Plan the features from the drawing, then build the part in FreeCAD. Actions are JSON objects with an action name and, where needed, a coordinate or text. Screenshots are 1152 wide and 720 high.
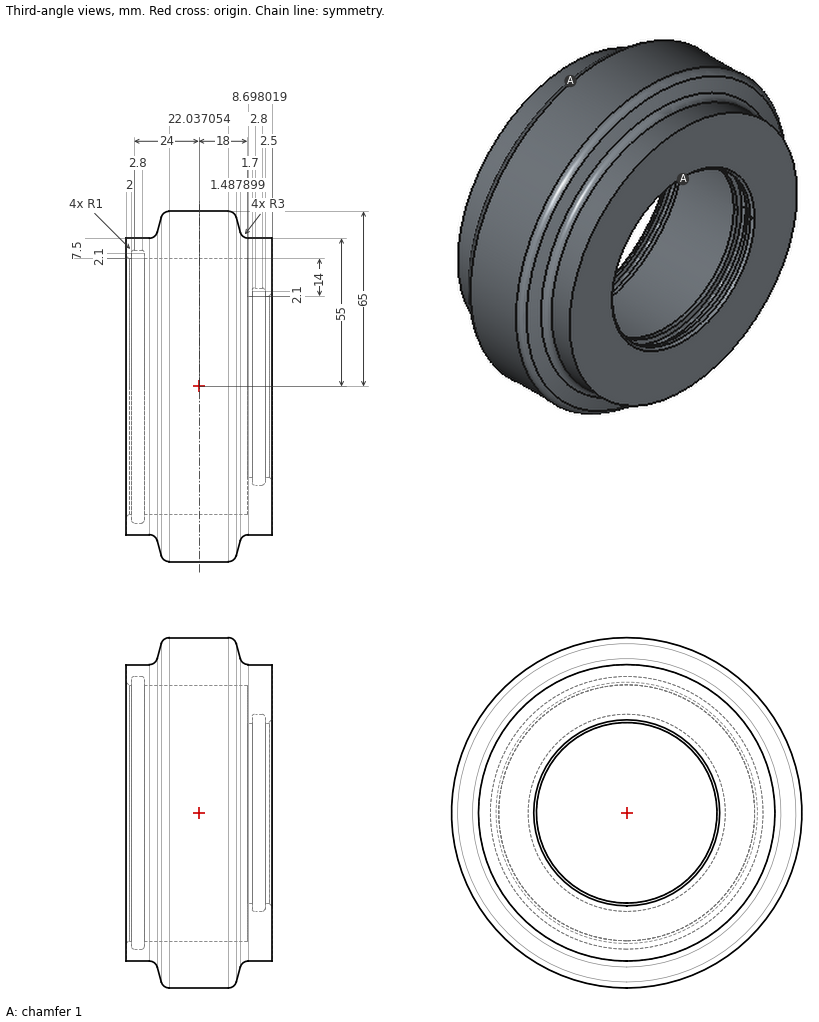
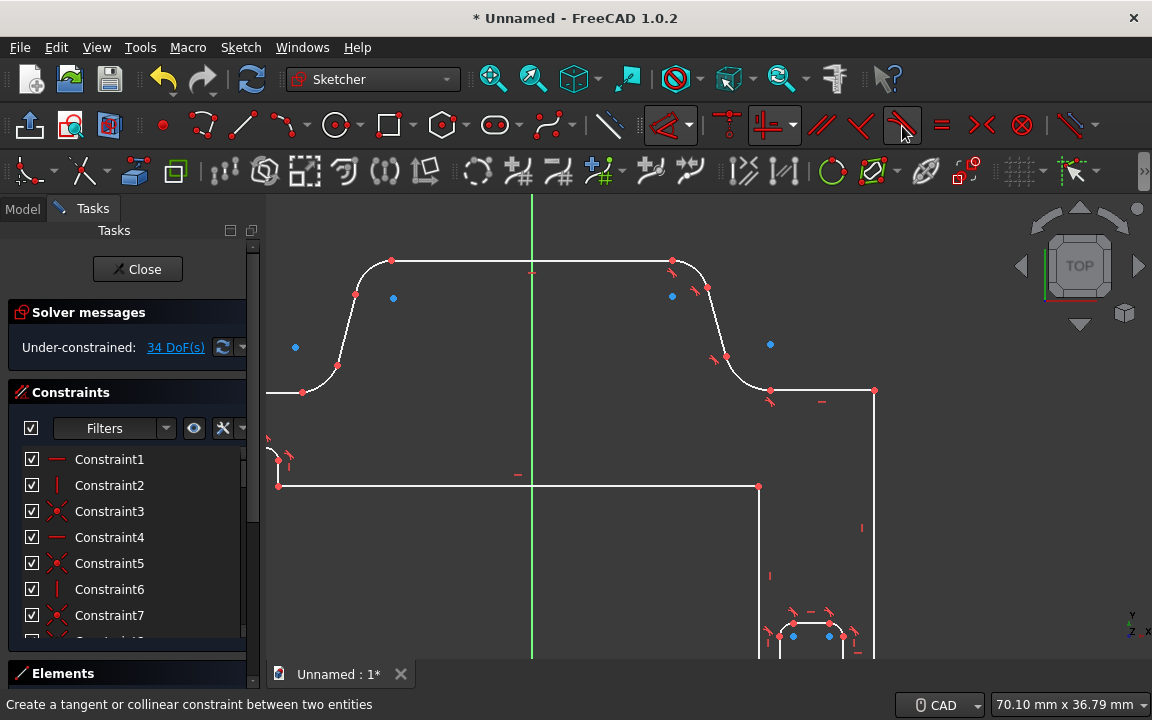
{"action": "left_click", "coordinate": [588, 261]}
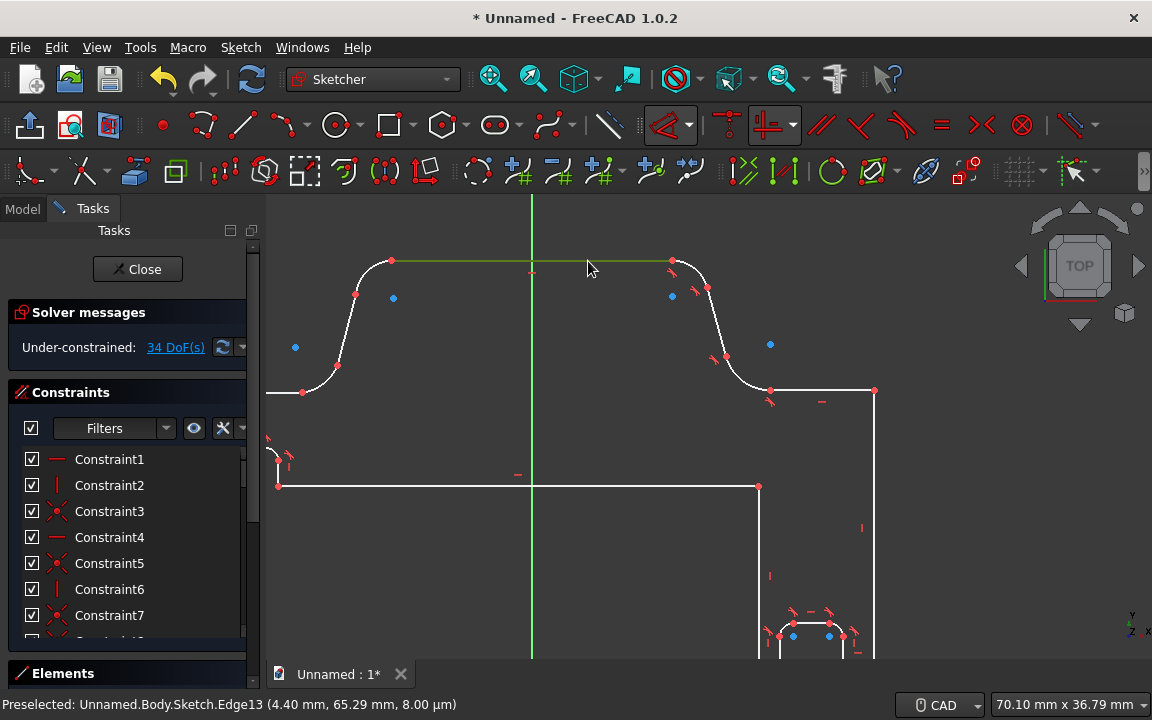
{"action": "left_click", "coordinate": [376, 265]}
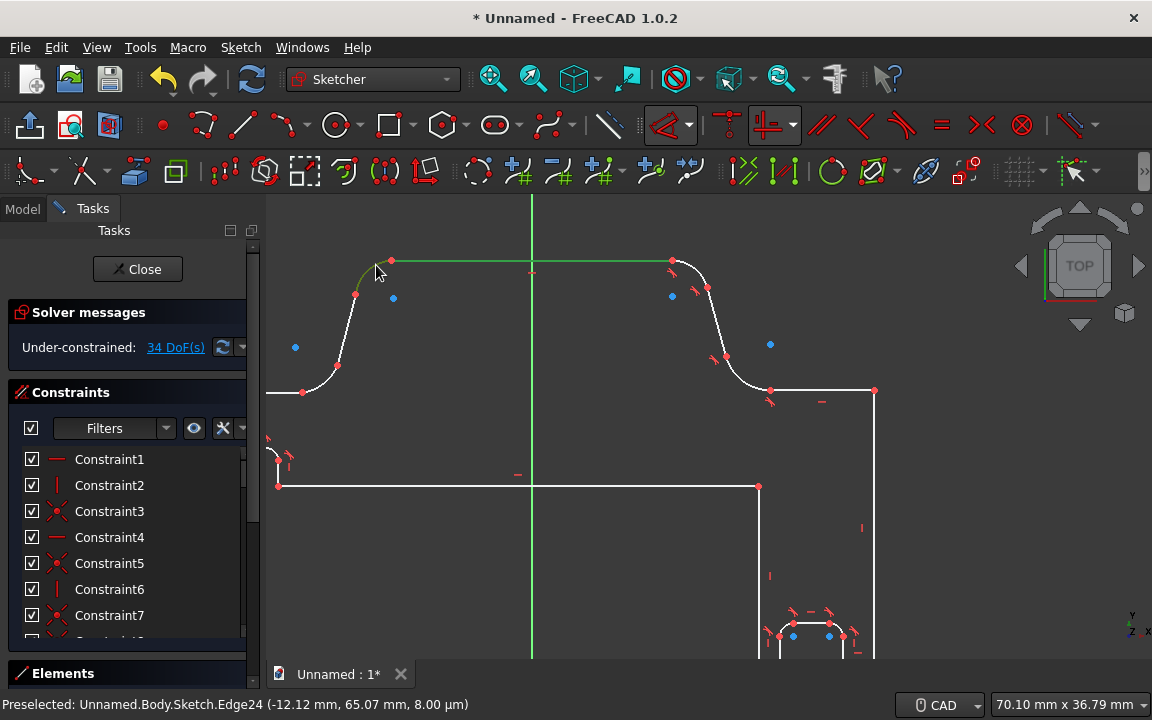
{"action": "key", "text": "t"}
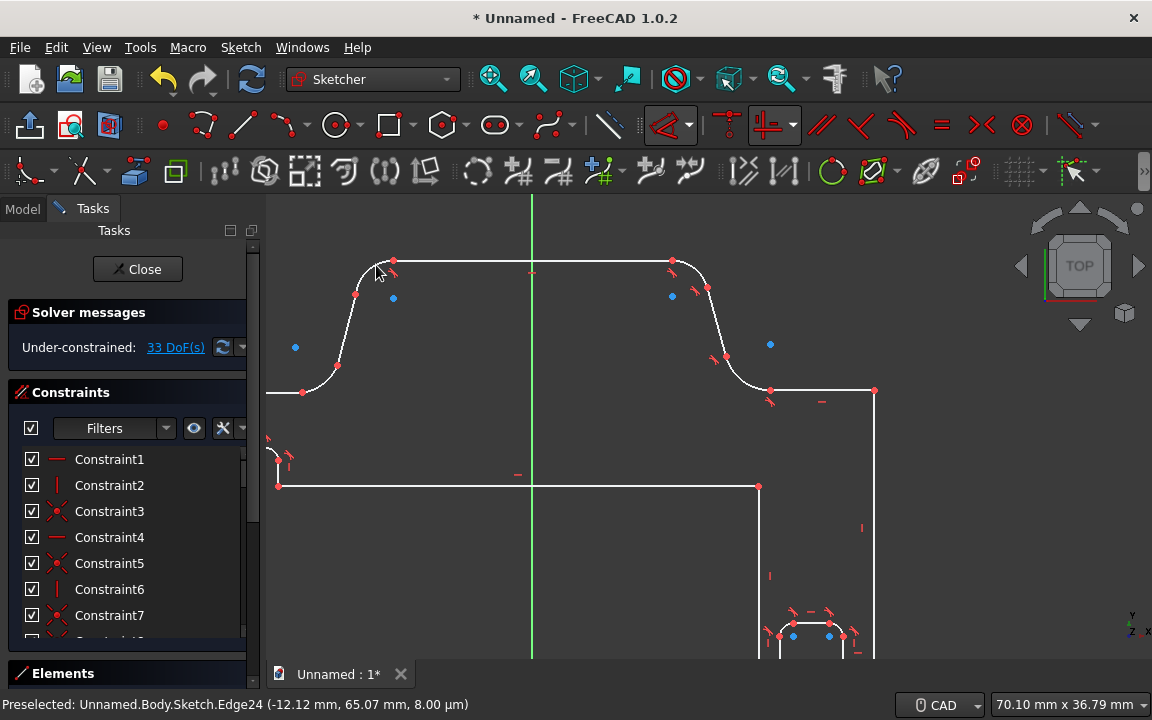
{"action": "left_click", "coordinate": [350, 316]}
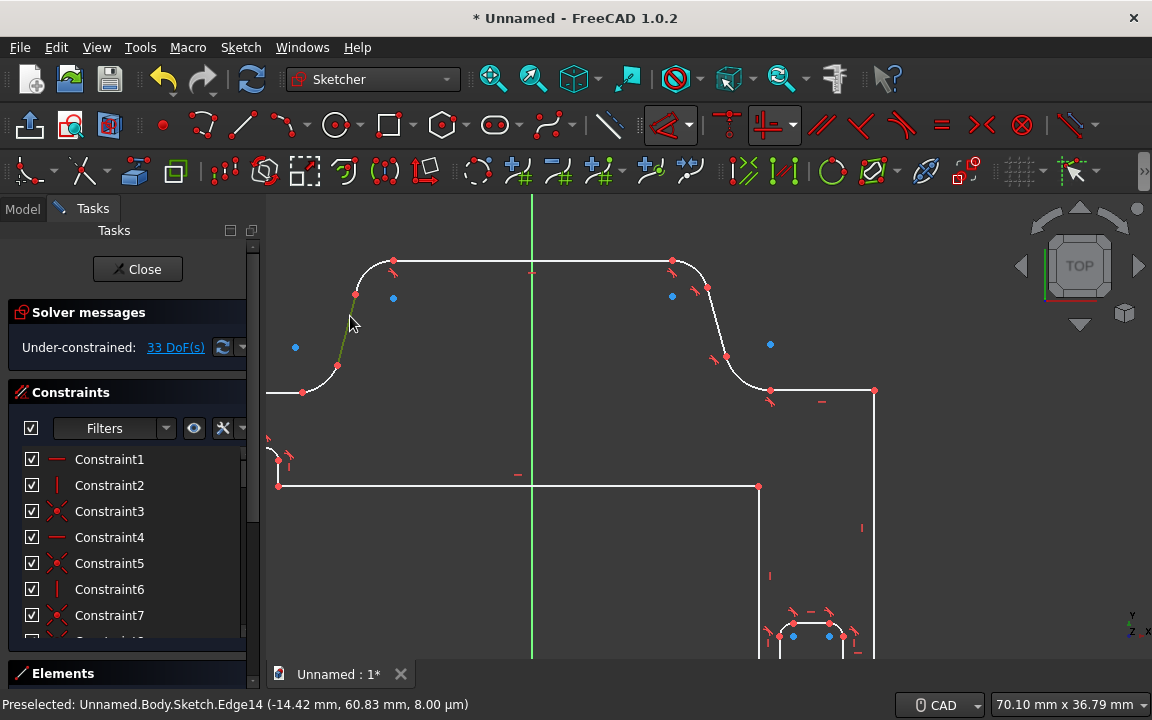
{"action": "left_click", "coordinate": [377, 264]}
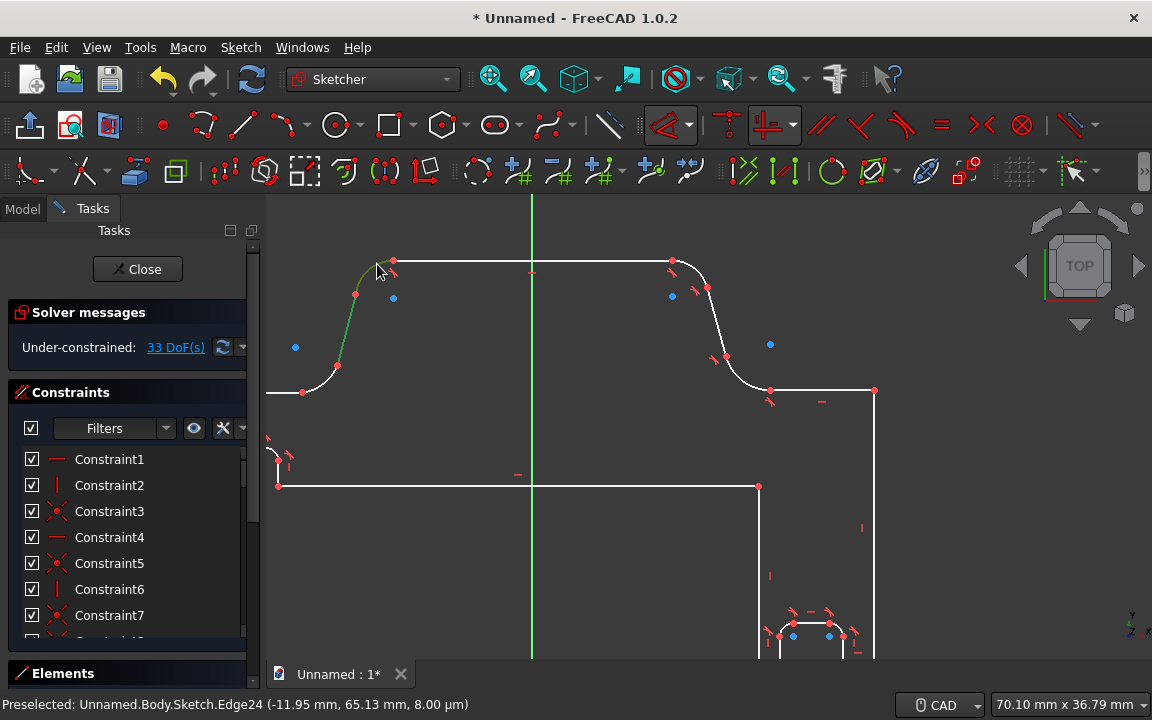
{"action": "key", "text": "t"}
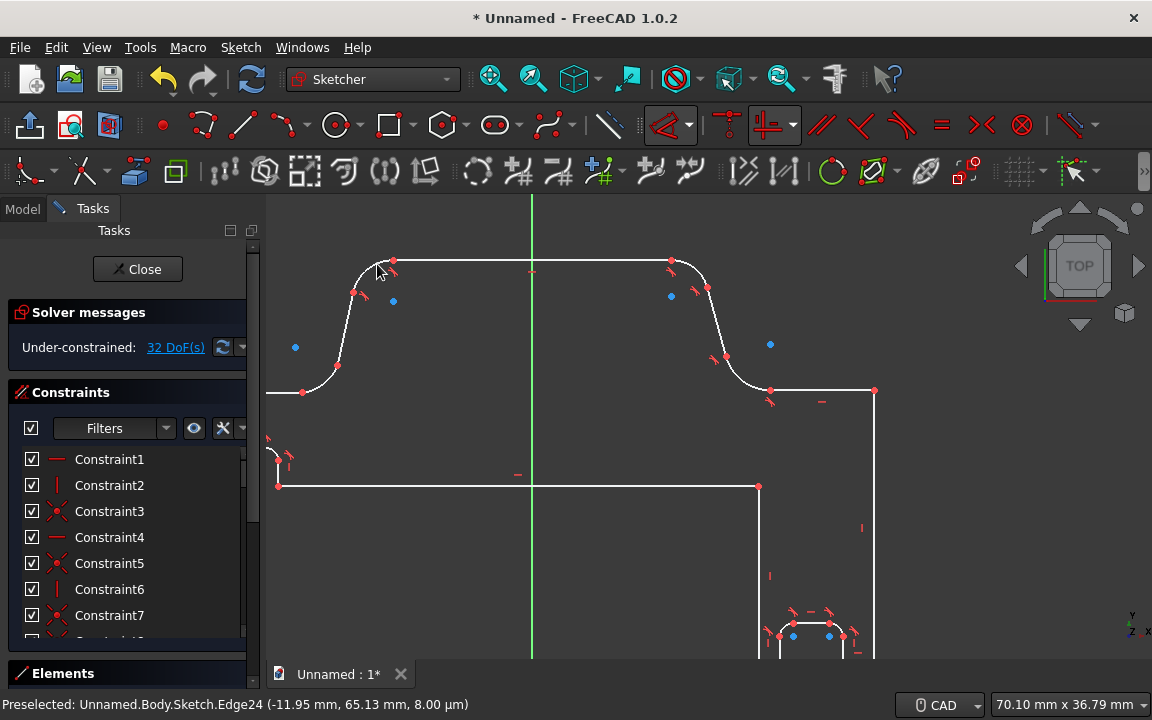
{"action": "left_click", "coordinate": [349, 315]}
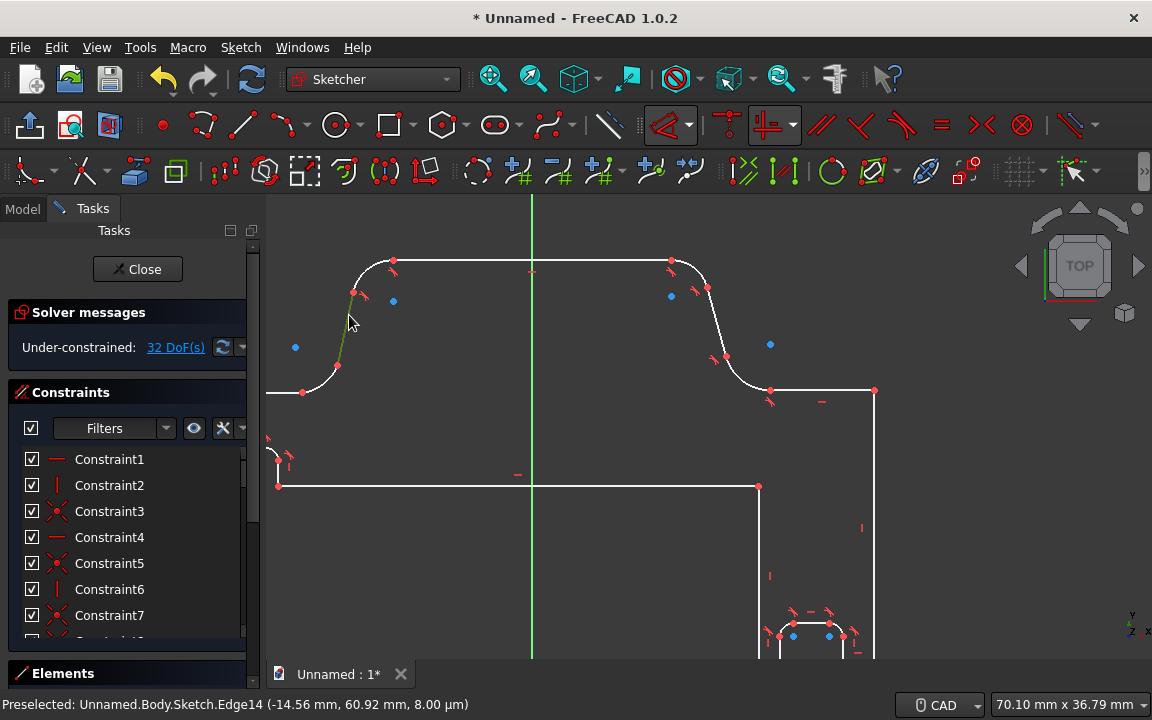
{"action": "left_click", "coordinate": [315, 389]}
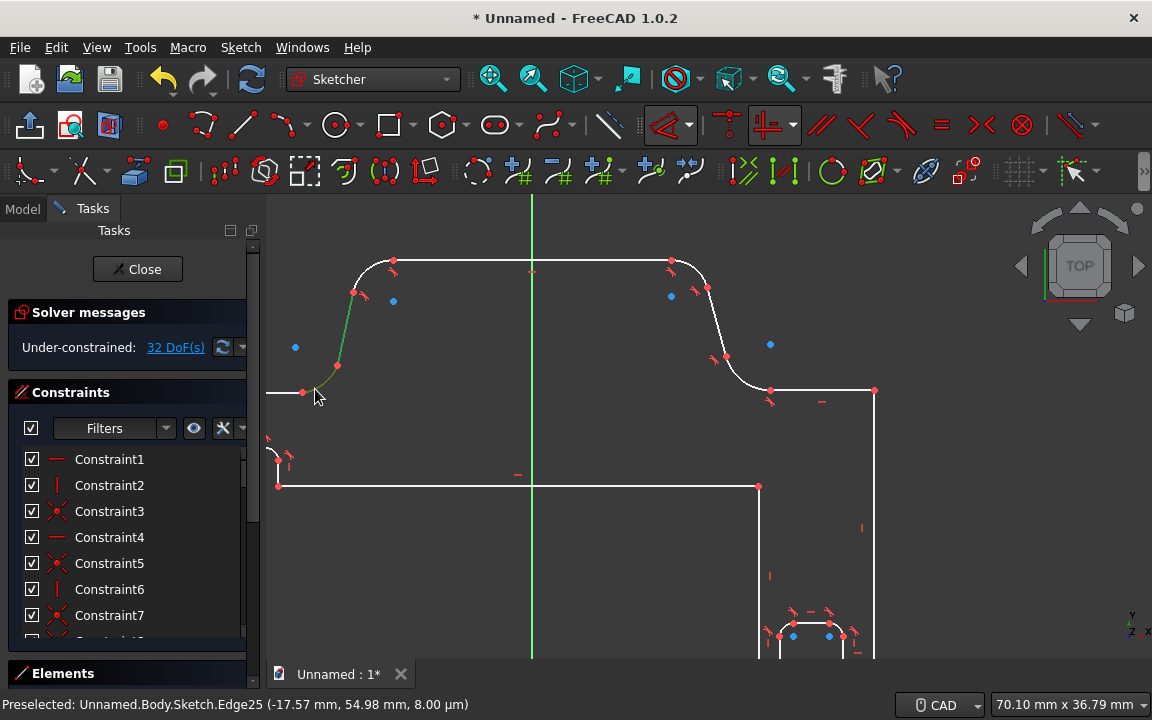
{"action": "left_click", "coordinate": [902, 126]}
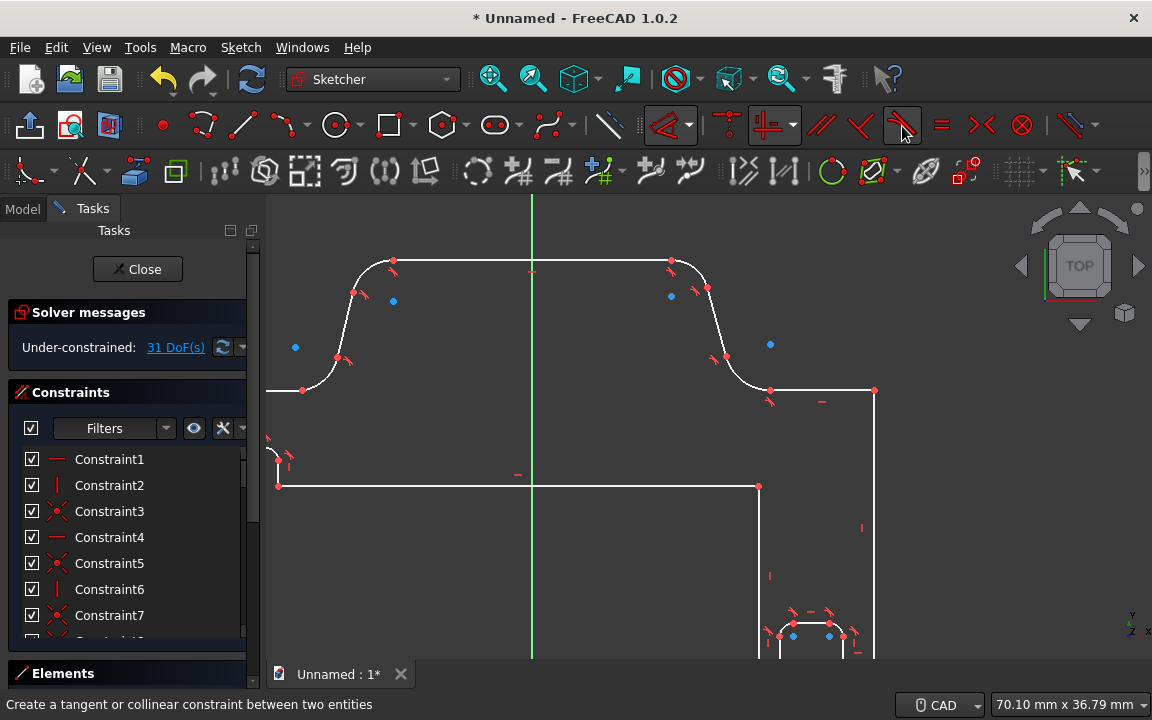
{"action": "scroll", "coordinate": [703, 282], "scroll_direction": "down", "scroll_amount": 5}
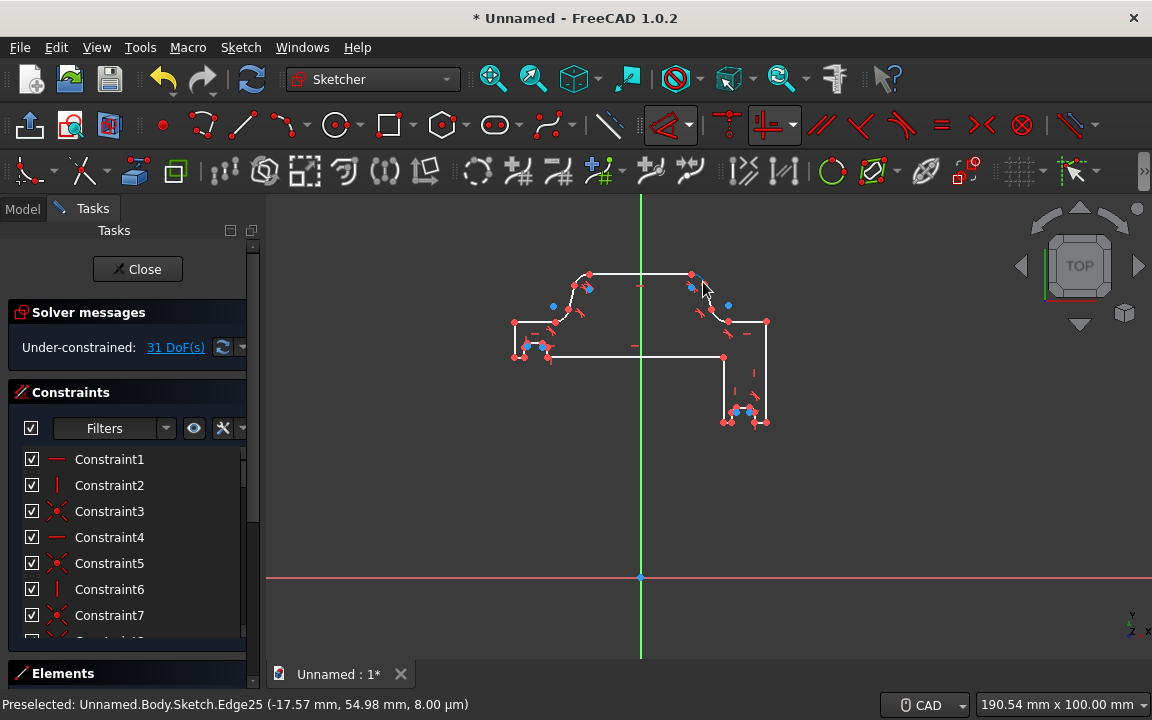
{"action": "left_click", "coordinate": [544, 322]}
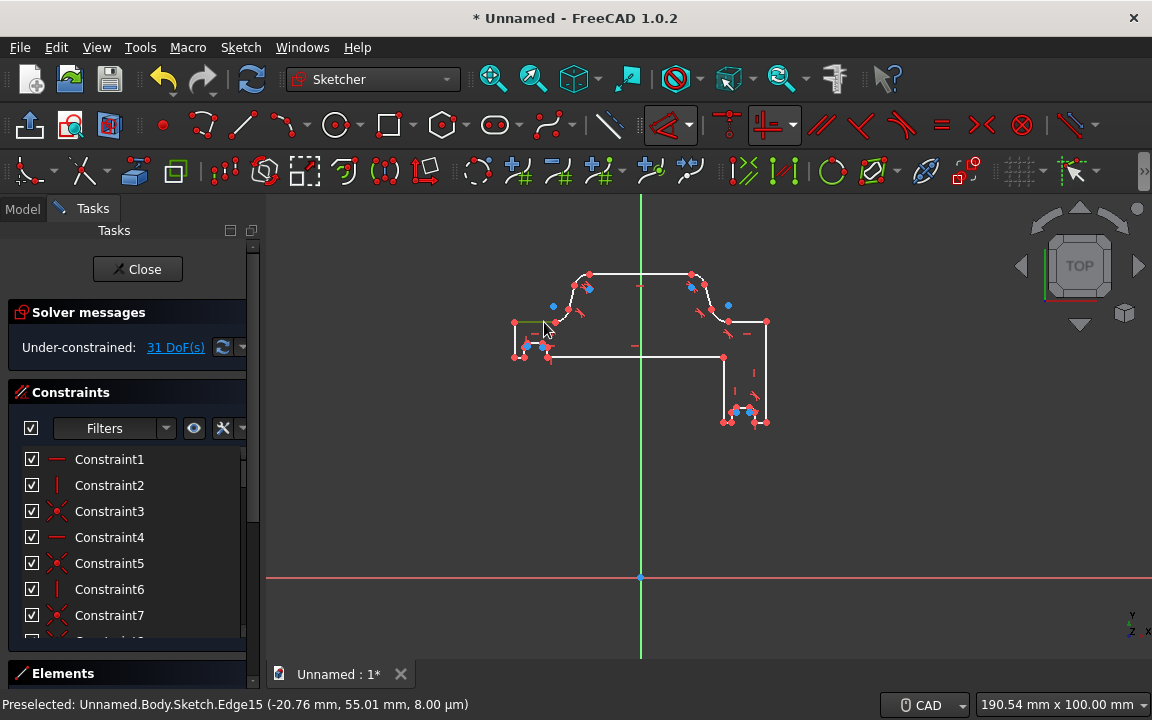
{"action": "scroll", "coordinate": [564, 318], "scroll_direction": "up", "scroll_amount": 2}